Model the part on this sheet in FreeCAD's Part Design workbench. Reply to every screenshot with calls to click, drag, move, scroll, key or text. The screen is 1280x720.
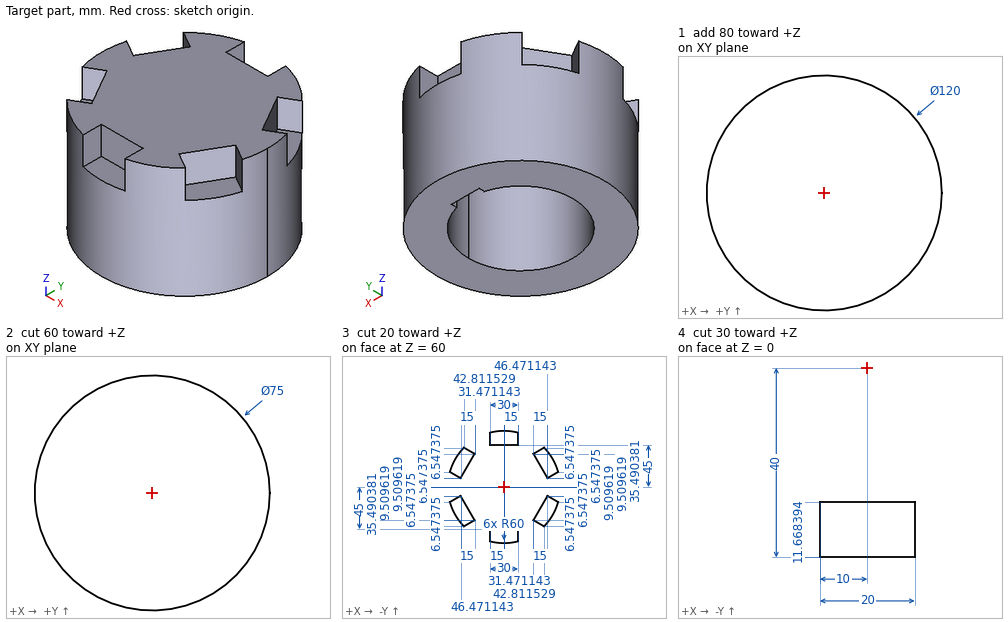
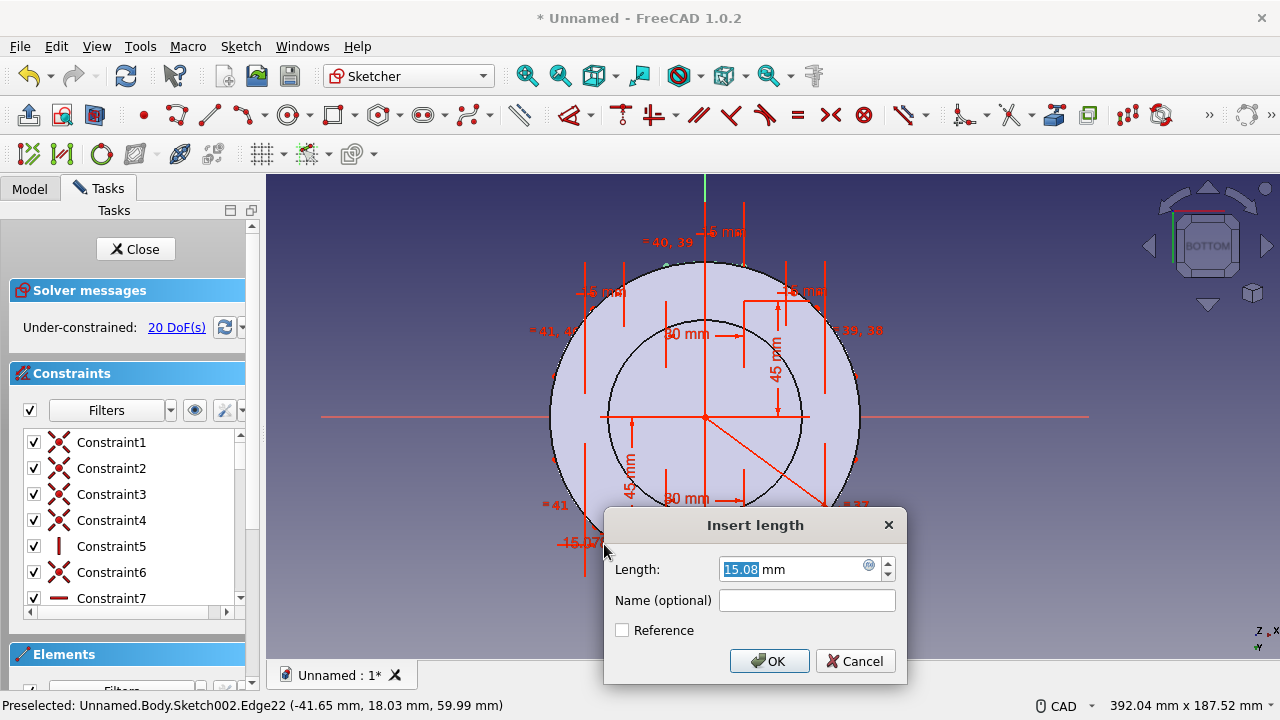
text(15)
key(Return)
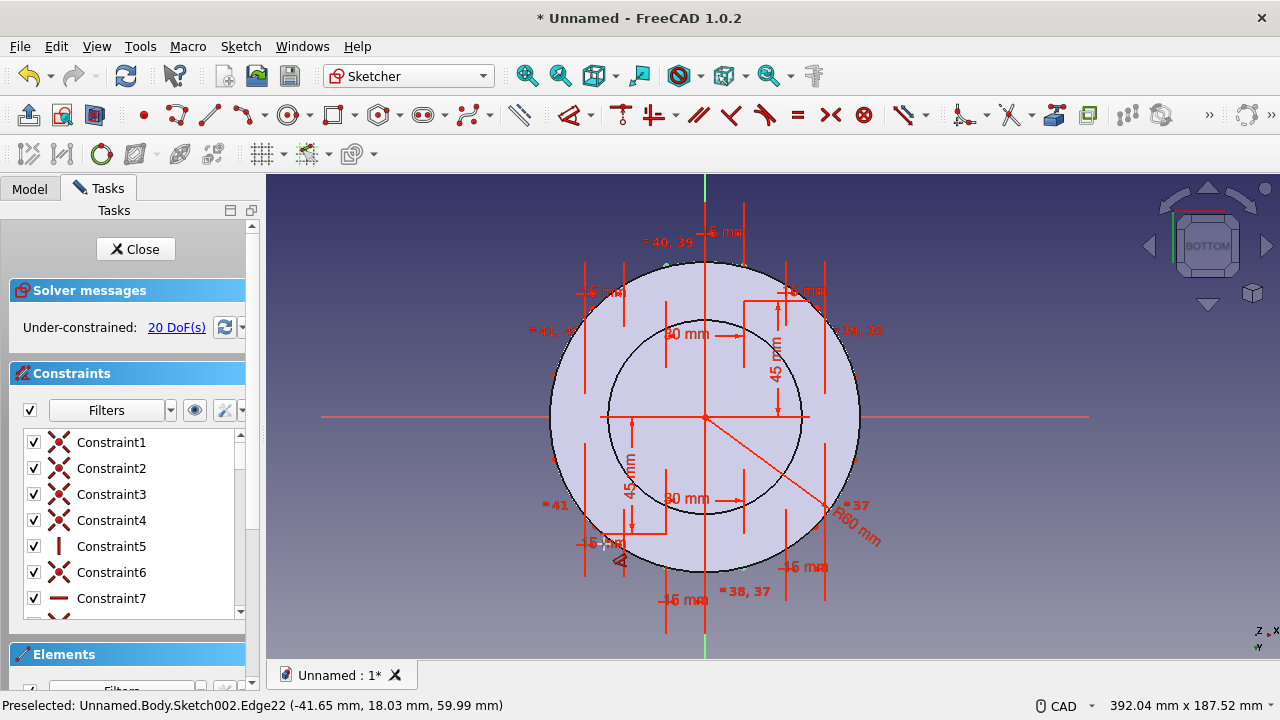
scroll(825, 443, up, 3)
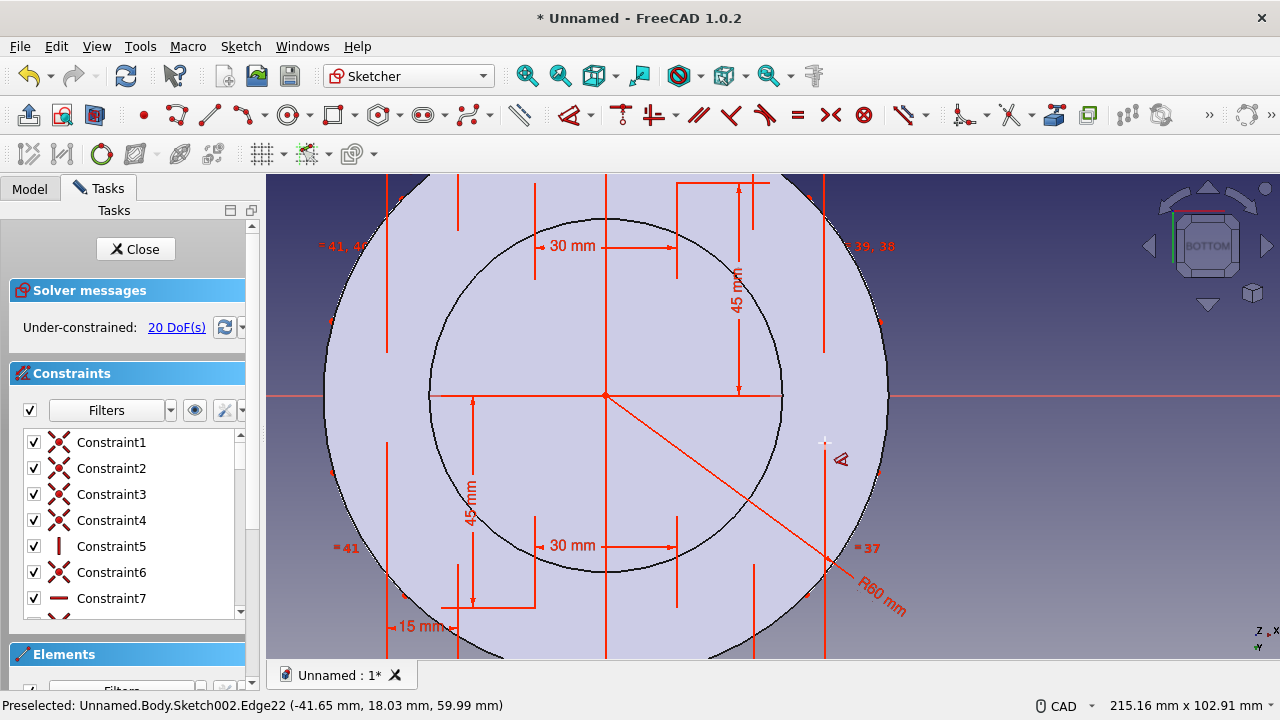
click(825, 442)
click(859, 419)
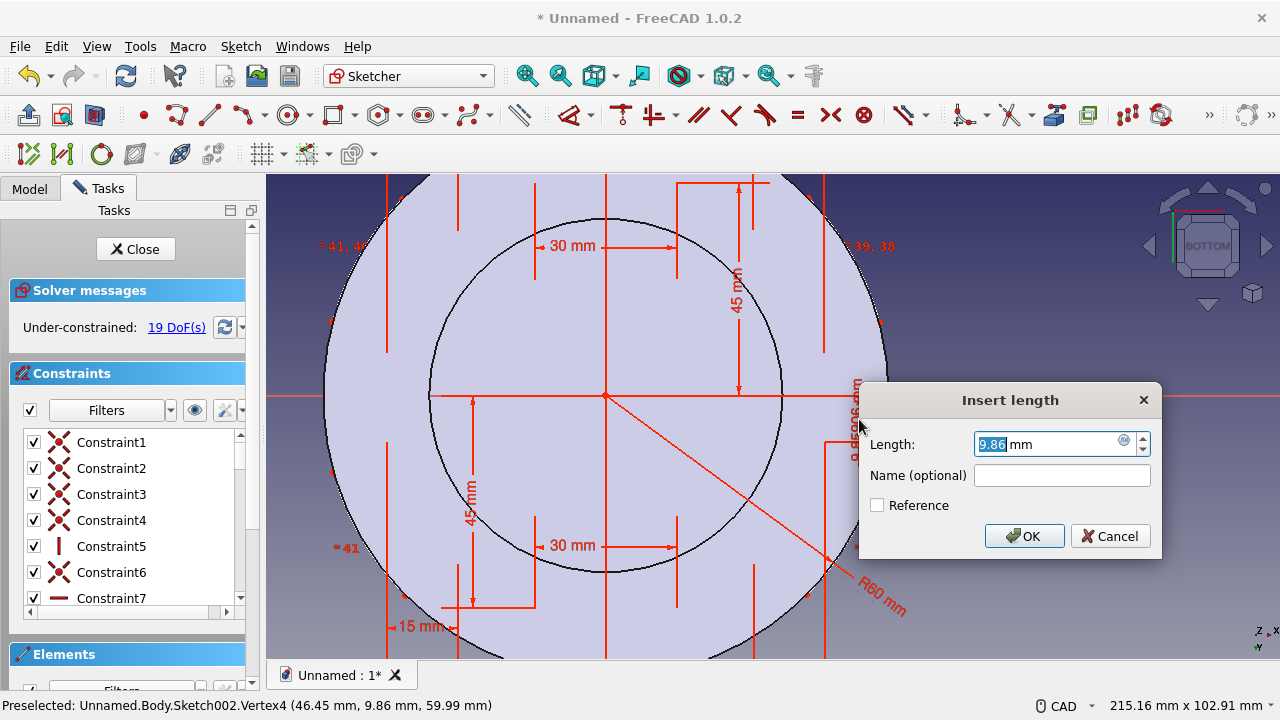
text(9.509619)
key(Return)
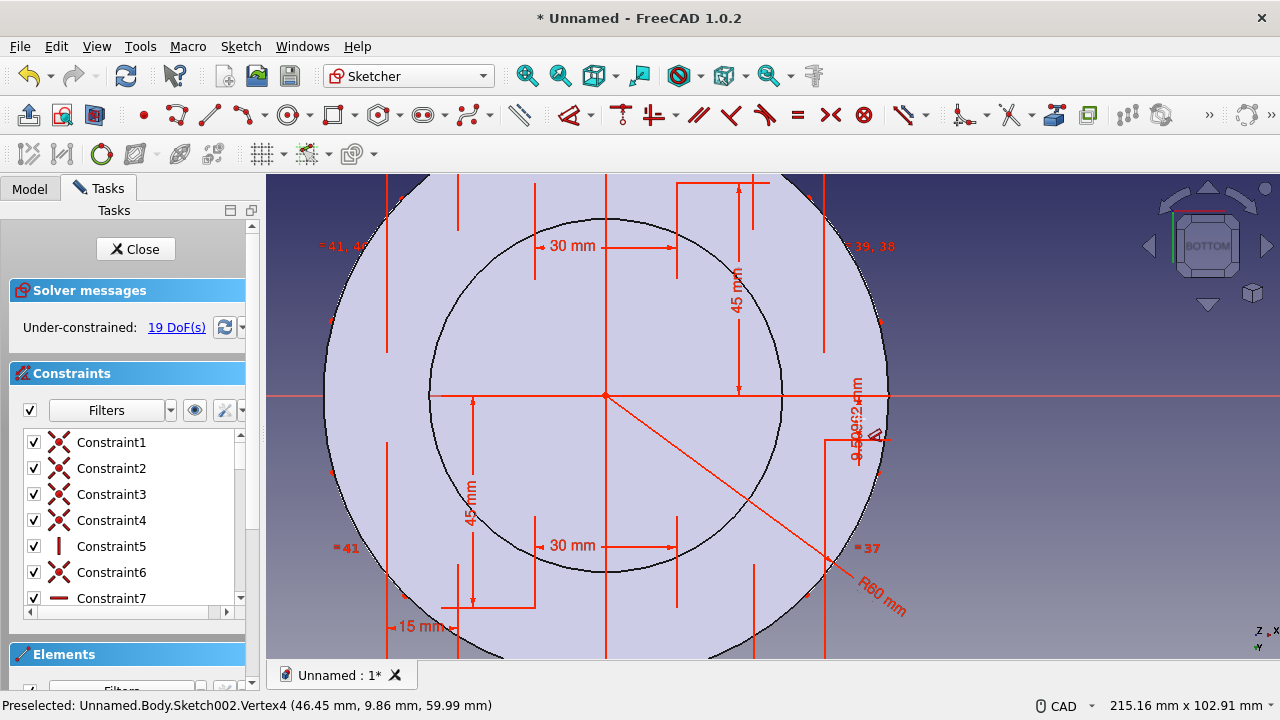
click(824, 353)
click(858, 374)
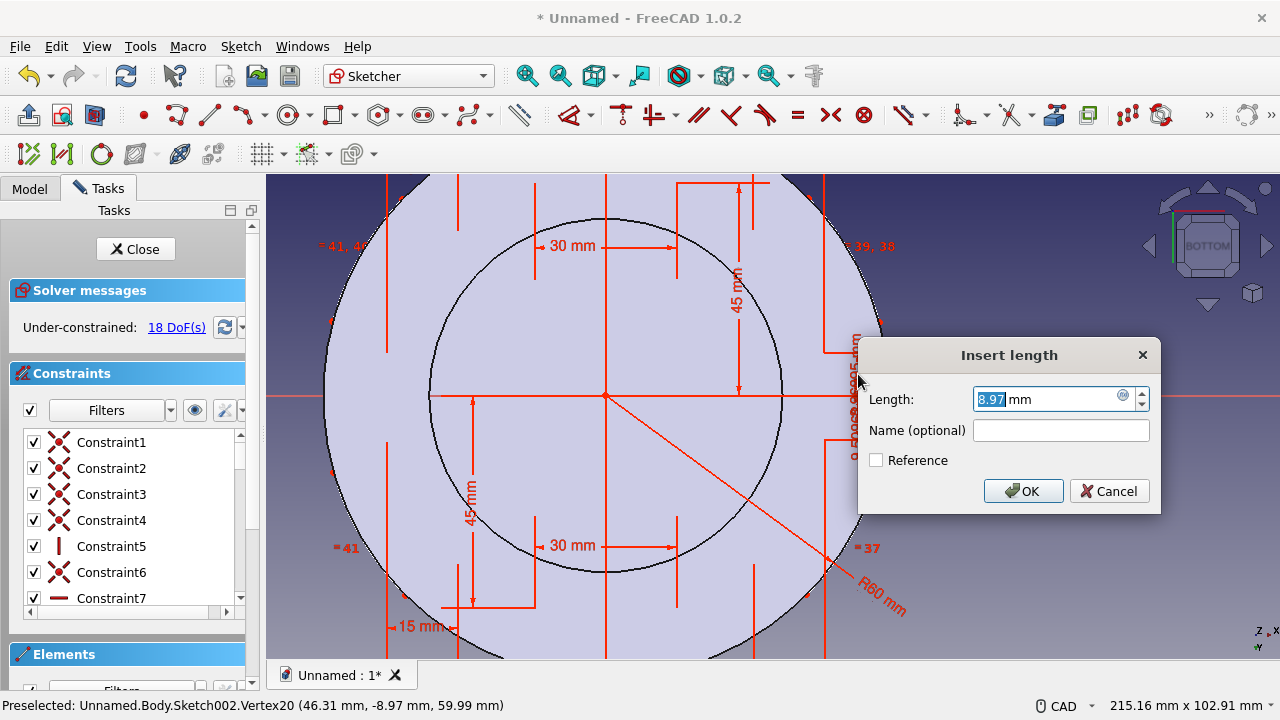
text(9.509619)
key(Return)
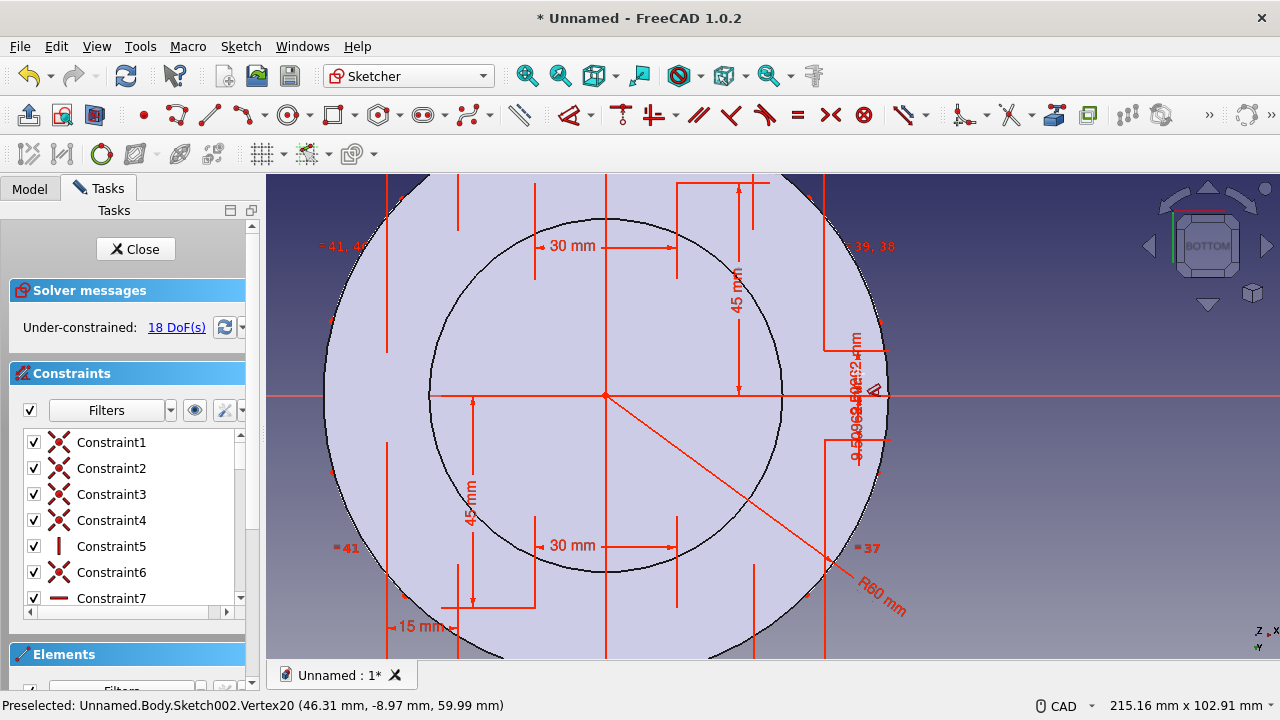
click(387, 353)
click(353, 374)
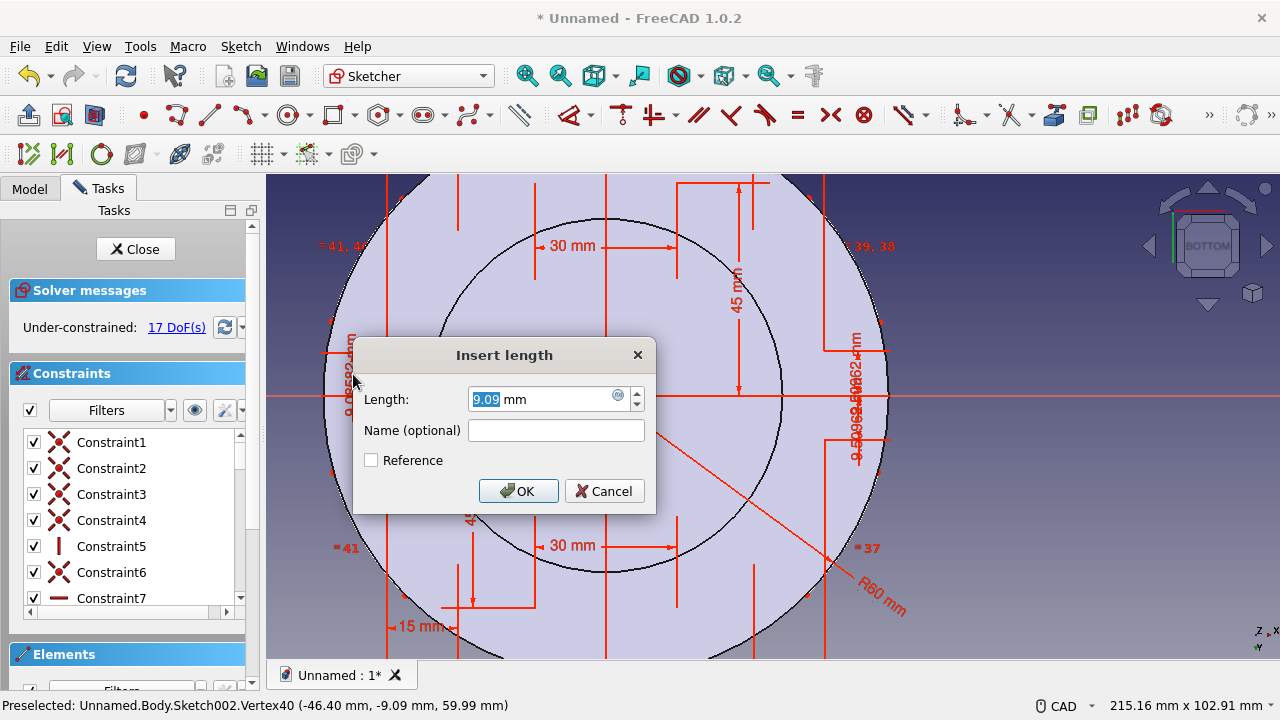
text(9.509619)
key(Return)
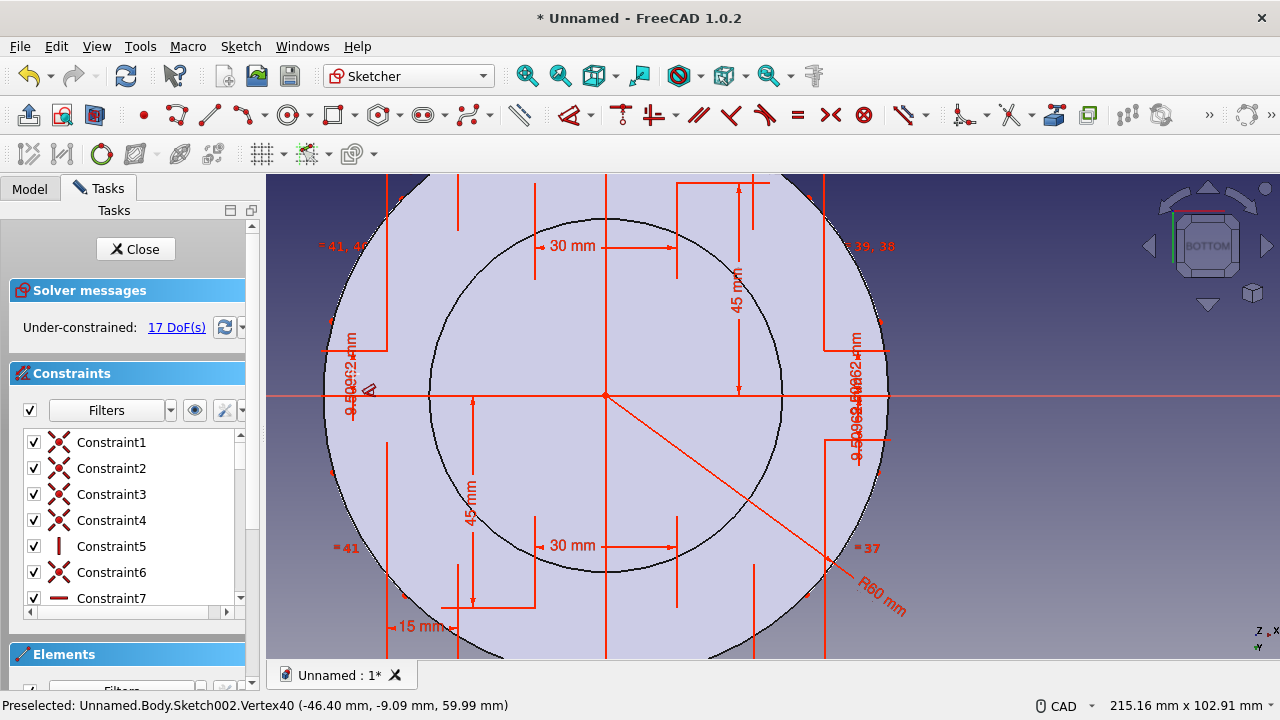
click(387, 442)
click(353, 419)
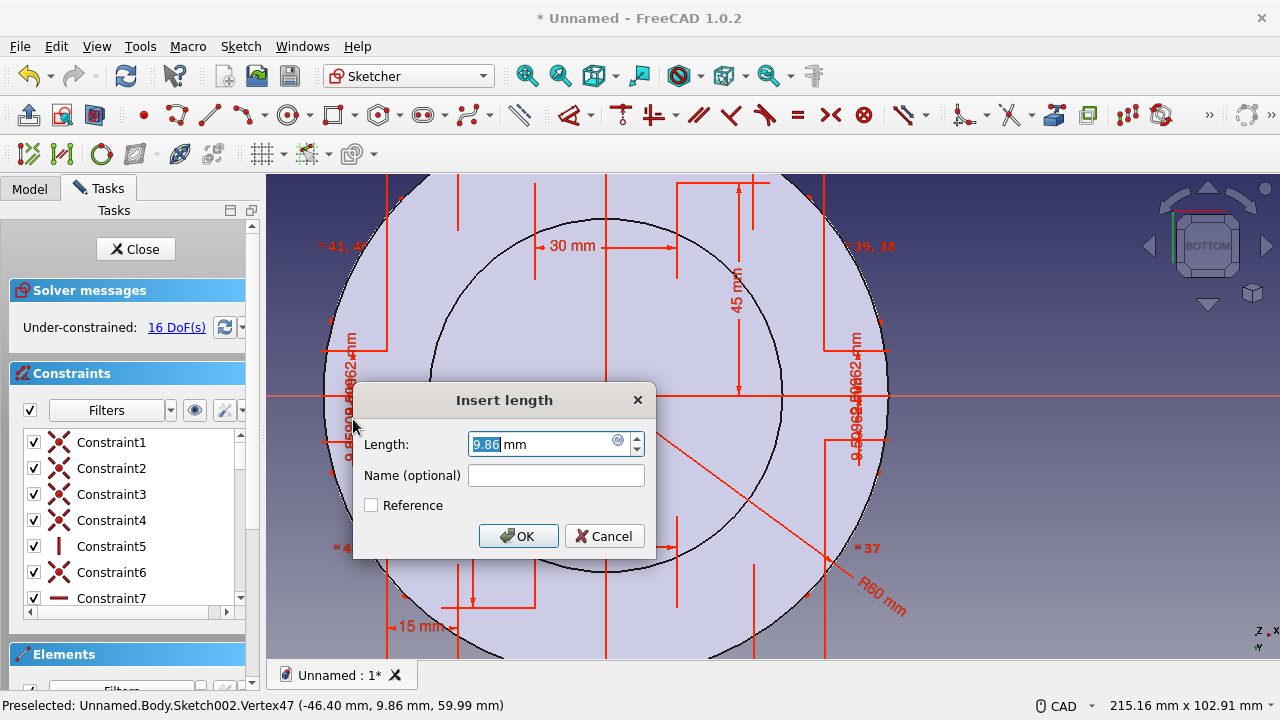
text(9.509619)
key(Return)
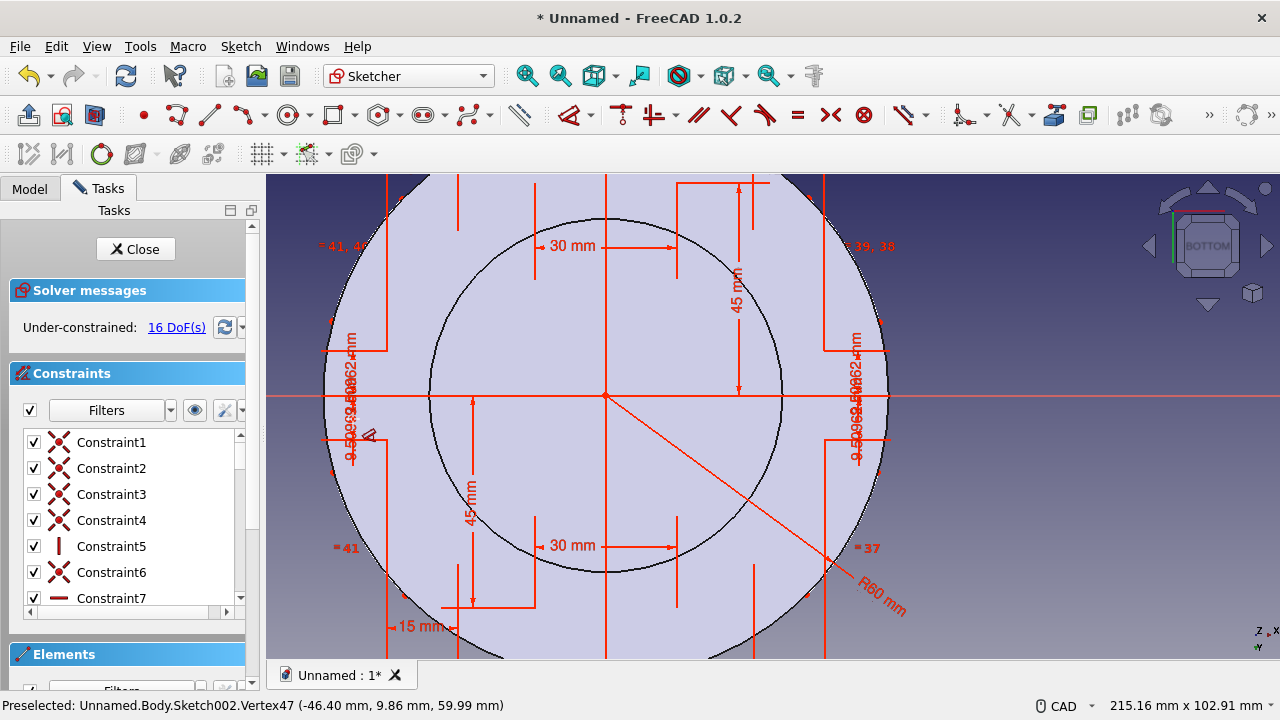
scroll(791, 586, up, 2)